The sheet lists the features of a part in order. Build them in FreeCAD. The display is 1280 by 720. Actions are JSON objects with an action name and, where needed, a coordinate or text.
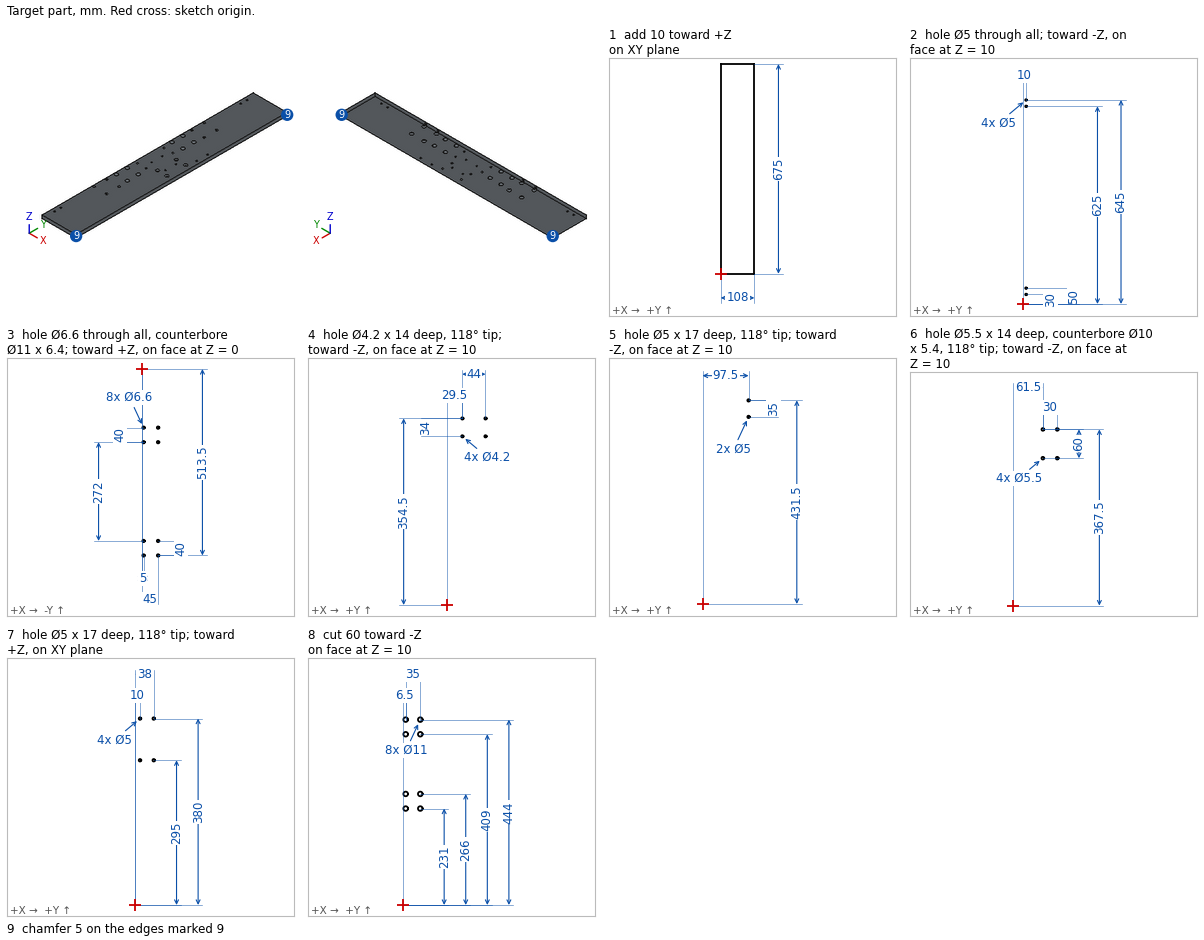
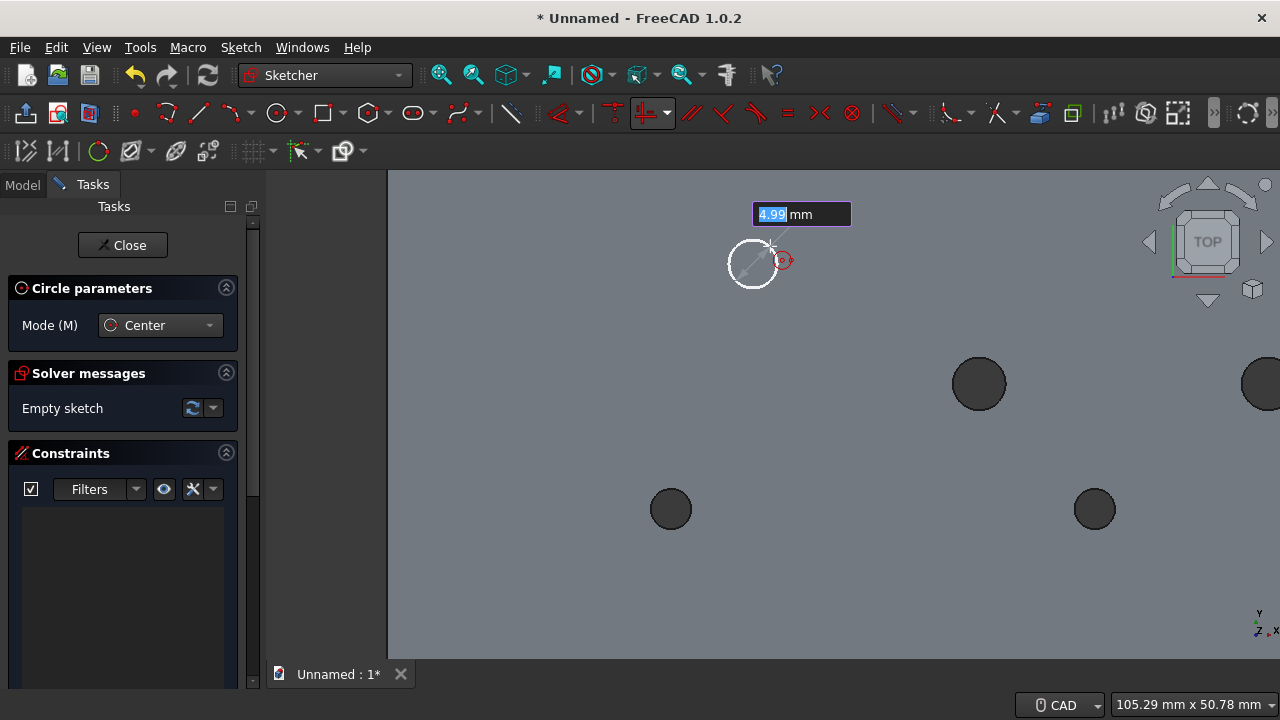
{"action": "type", "text": "5"}
{"action": "key", "text": "Return"}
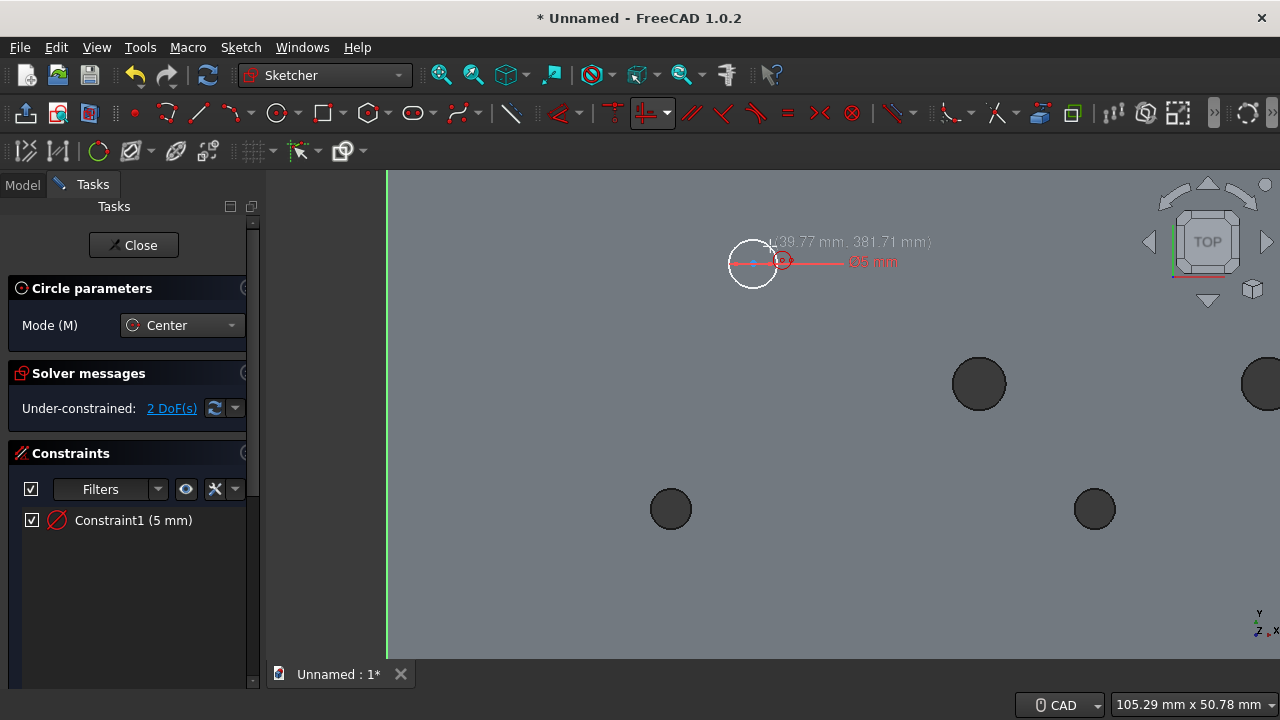
{"action": "left_click", "coordinate": [483, 263]}
{"action": "mouse_move", "coordinate": [500, 246]}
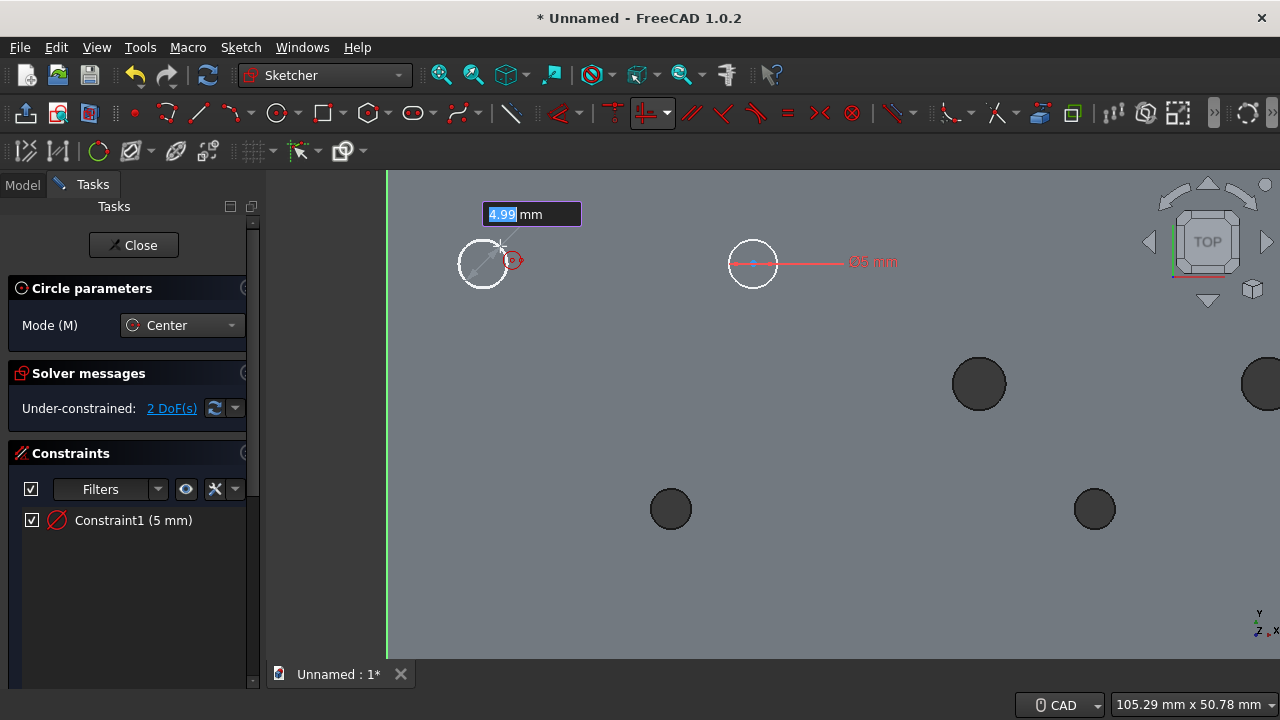
{"action": "type", "text": "5"}
{"action": "key", "text": "Return"}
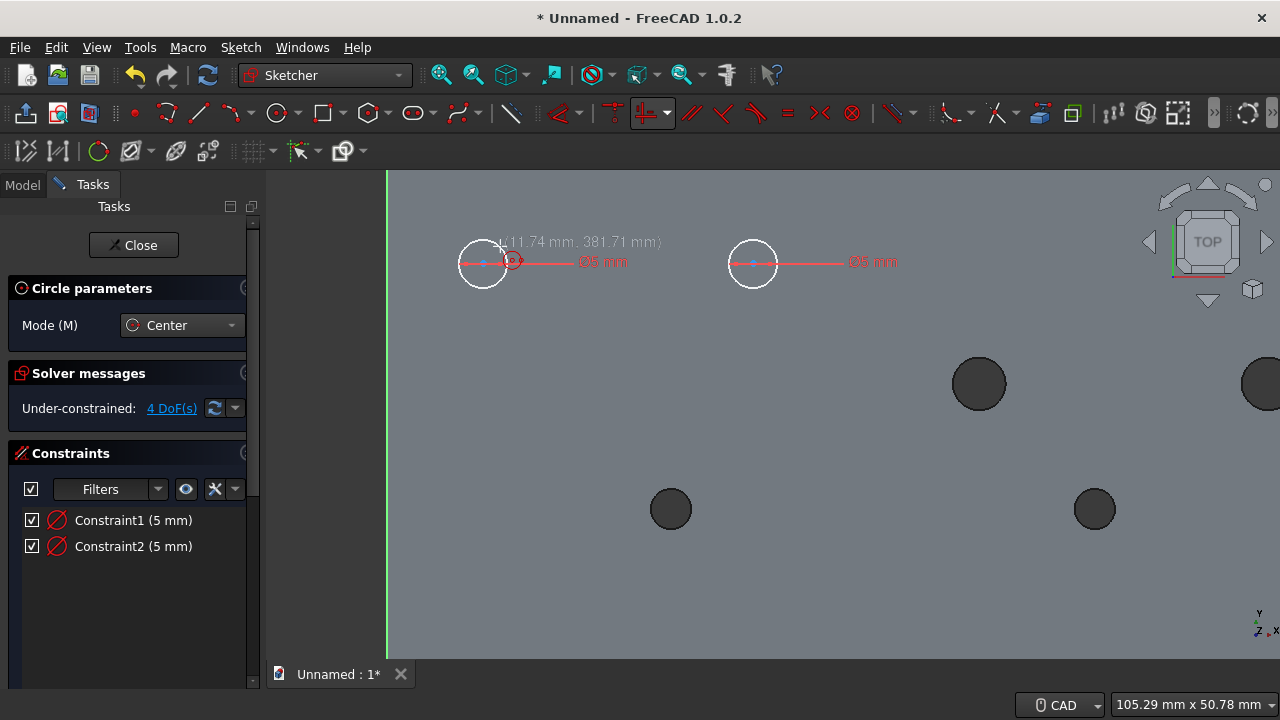
{"action": "scroll", "coordinate": [755, 264], "scroll_direction": "down", "scroll_amount": 5}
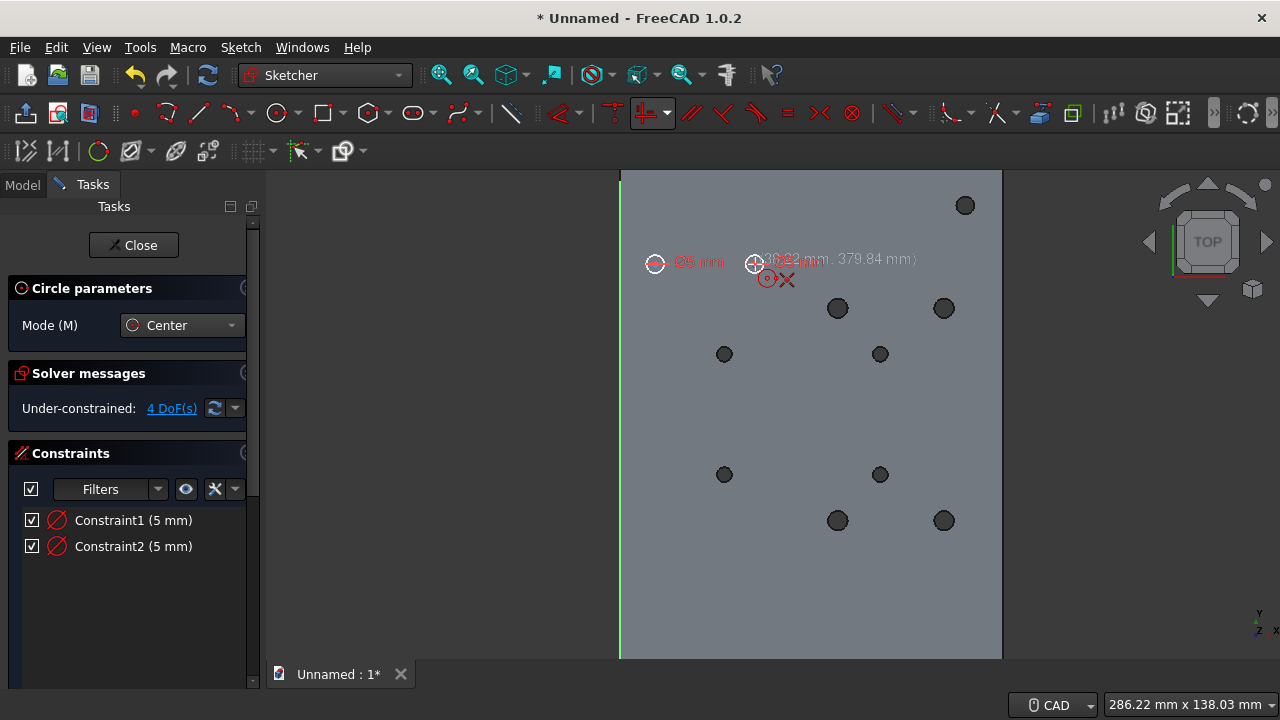
{"action": "scroll", "coordinate": [755, 565], "scroll_direction": "up", "scroll_amount": 5}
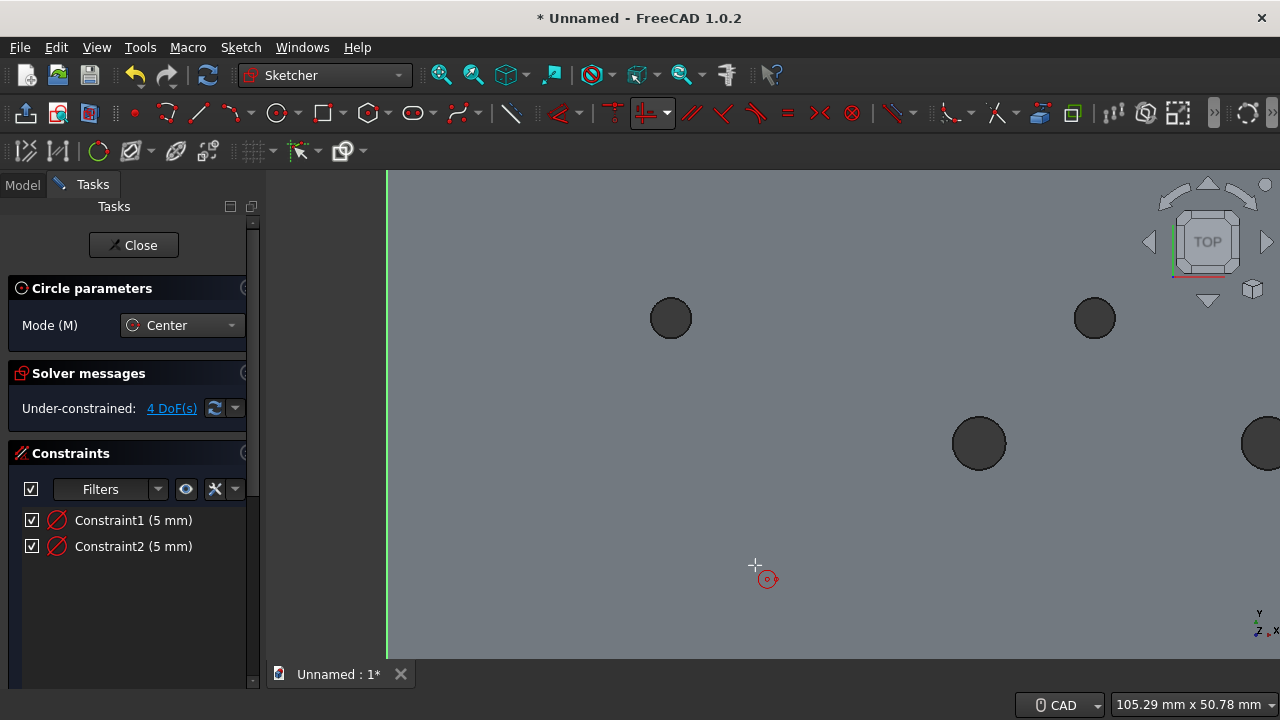
{"action": "left_click", "coordinate": [753, 564]}
{"action": "mouse_move", "coordinate": [770, 547]}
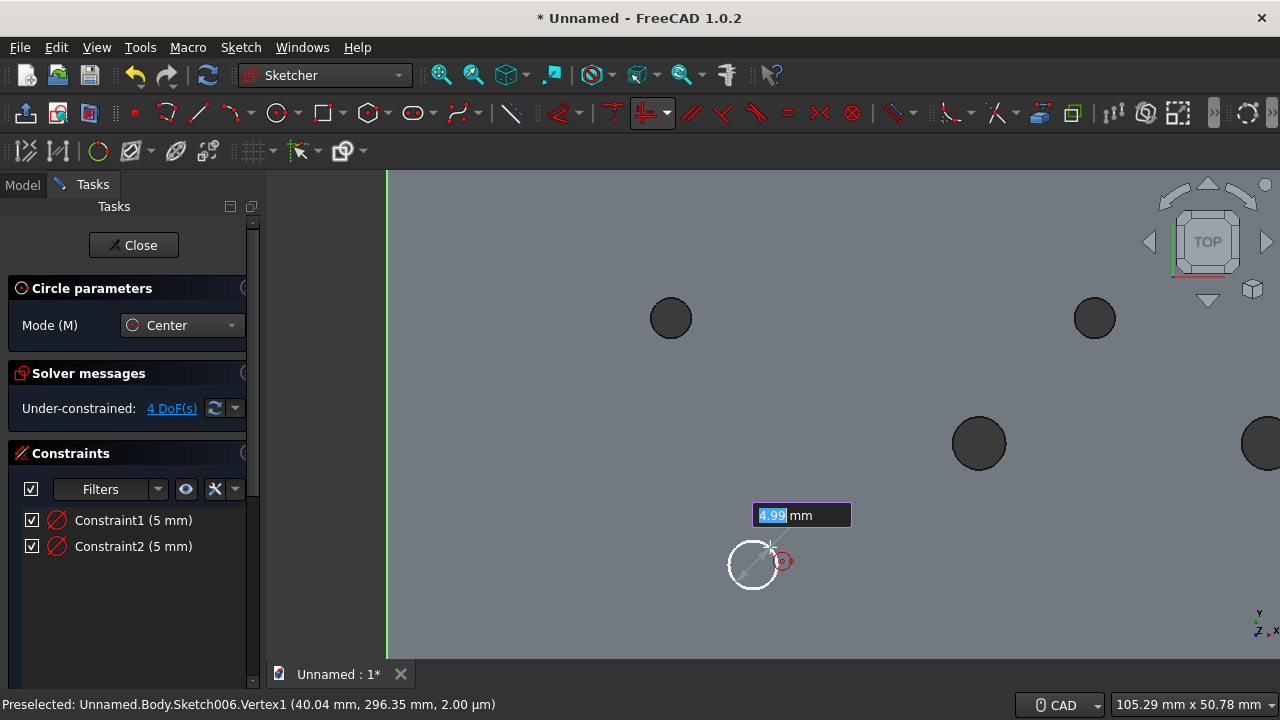
{"action": "type", "text": "5"}
{"action": "key", "text": "Return"}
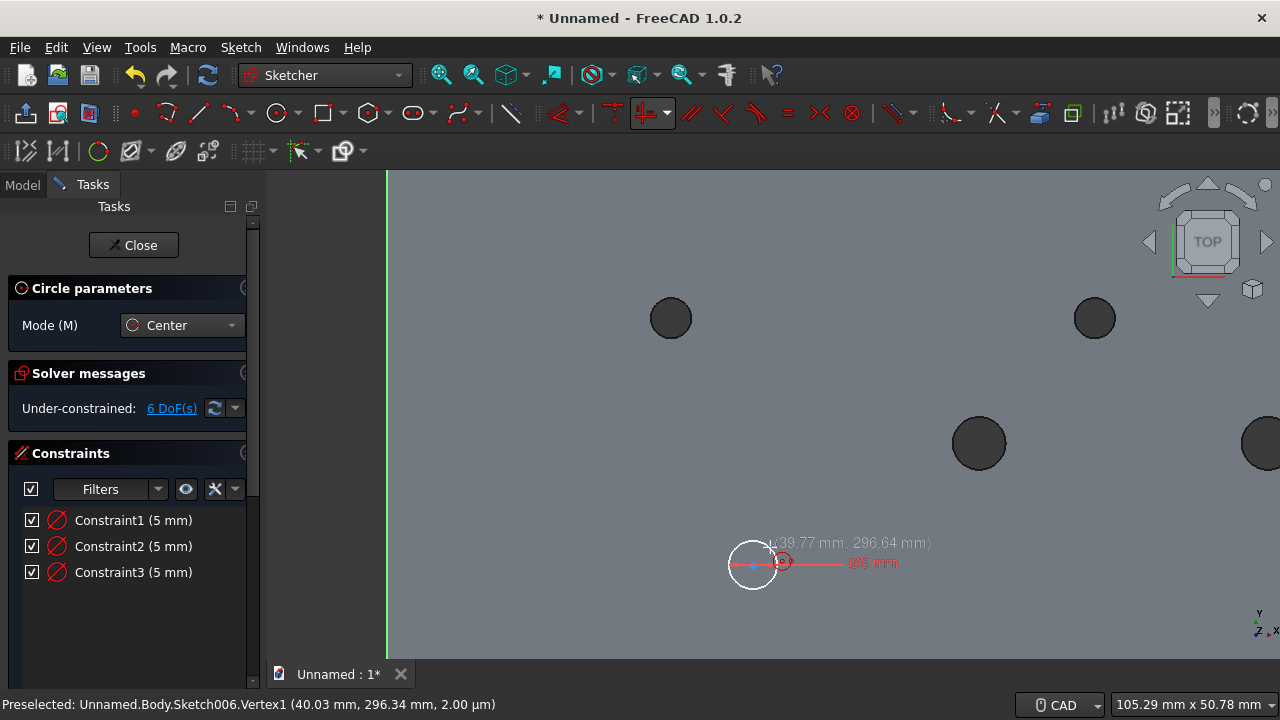
{"action": "left_click", "coordinate": [483, 564]}
{"action": "mouse_move", "coordinate": [500, 547]}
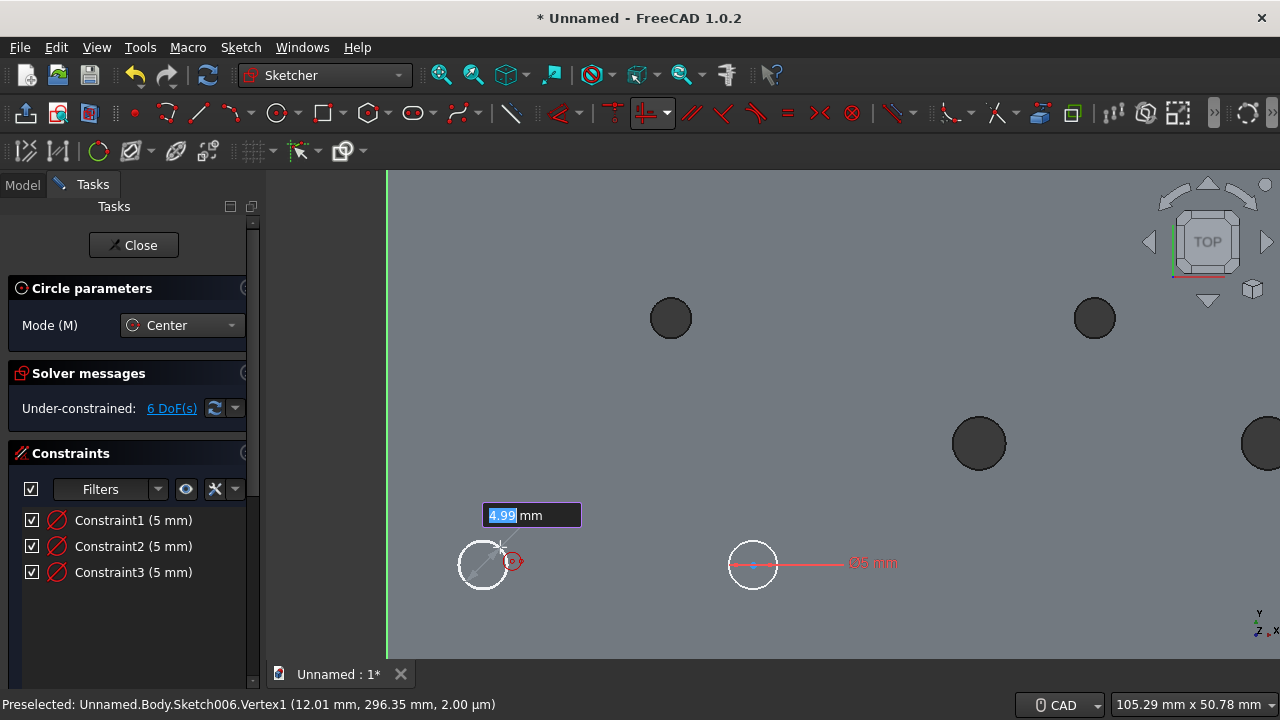
{"action": "type", "text": "5"}
{"action": "key", "text": "Return"}
{"action": "key", "text": "Escape"}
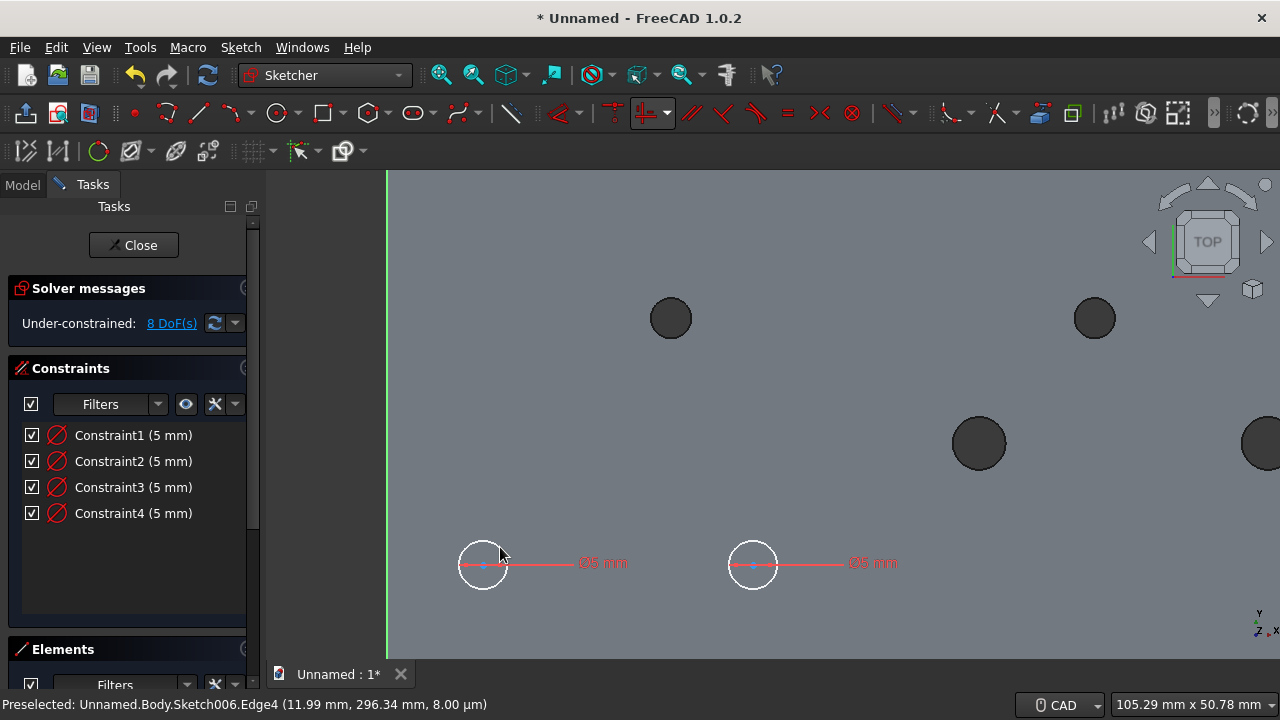
{"action": "scroll", "coordinate": [755, 566], "scroll_direction": "down", "scroll_amount": 5}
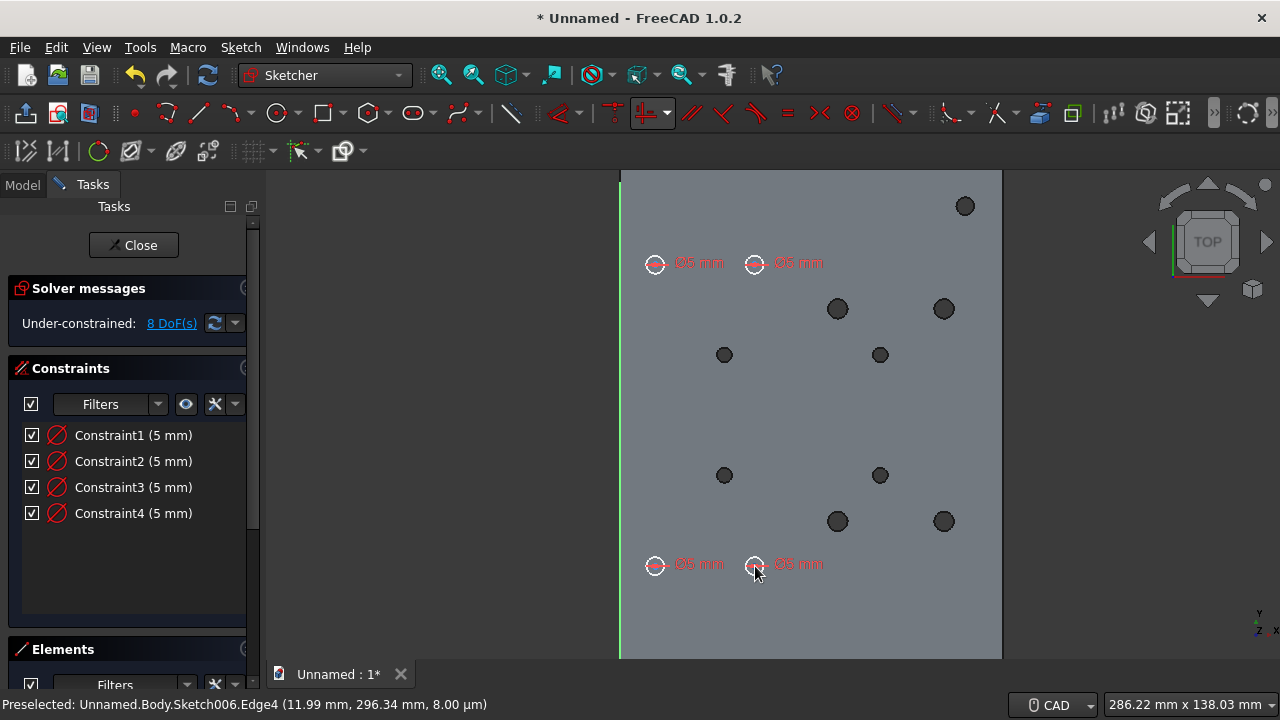
{"action": "left_click", "coordinate": [755, 265]}